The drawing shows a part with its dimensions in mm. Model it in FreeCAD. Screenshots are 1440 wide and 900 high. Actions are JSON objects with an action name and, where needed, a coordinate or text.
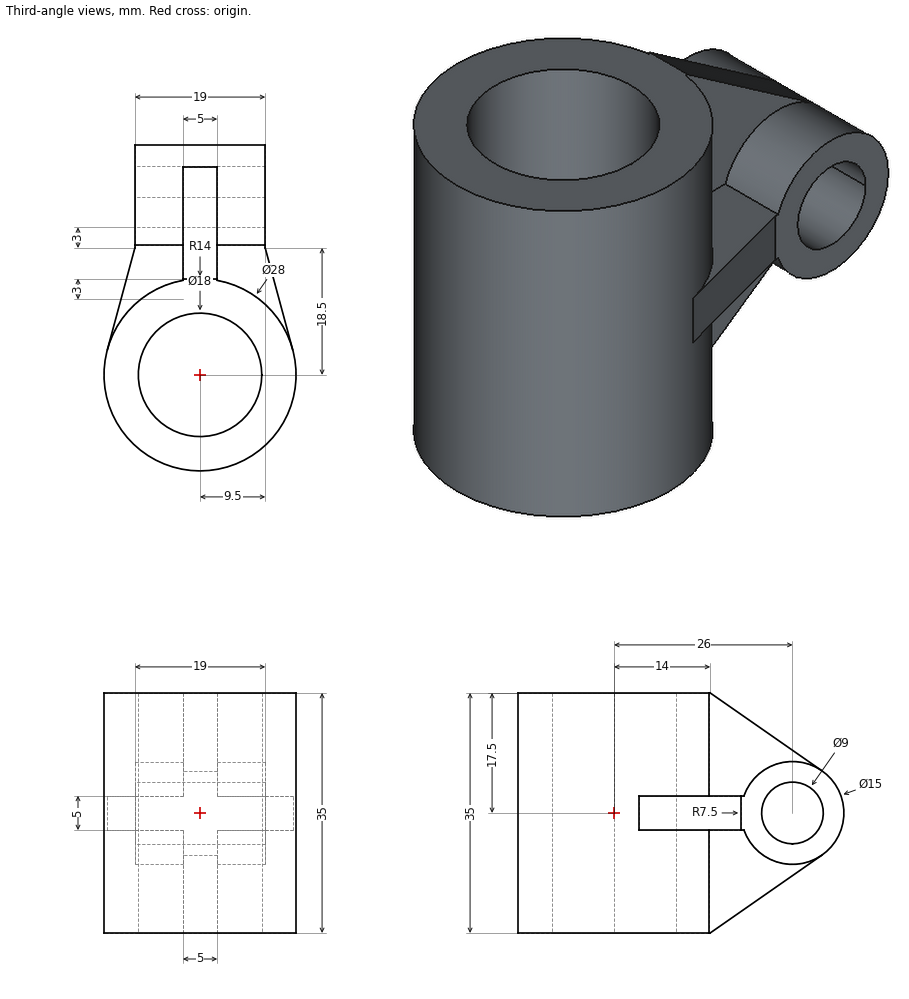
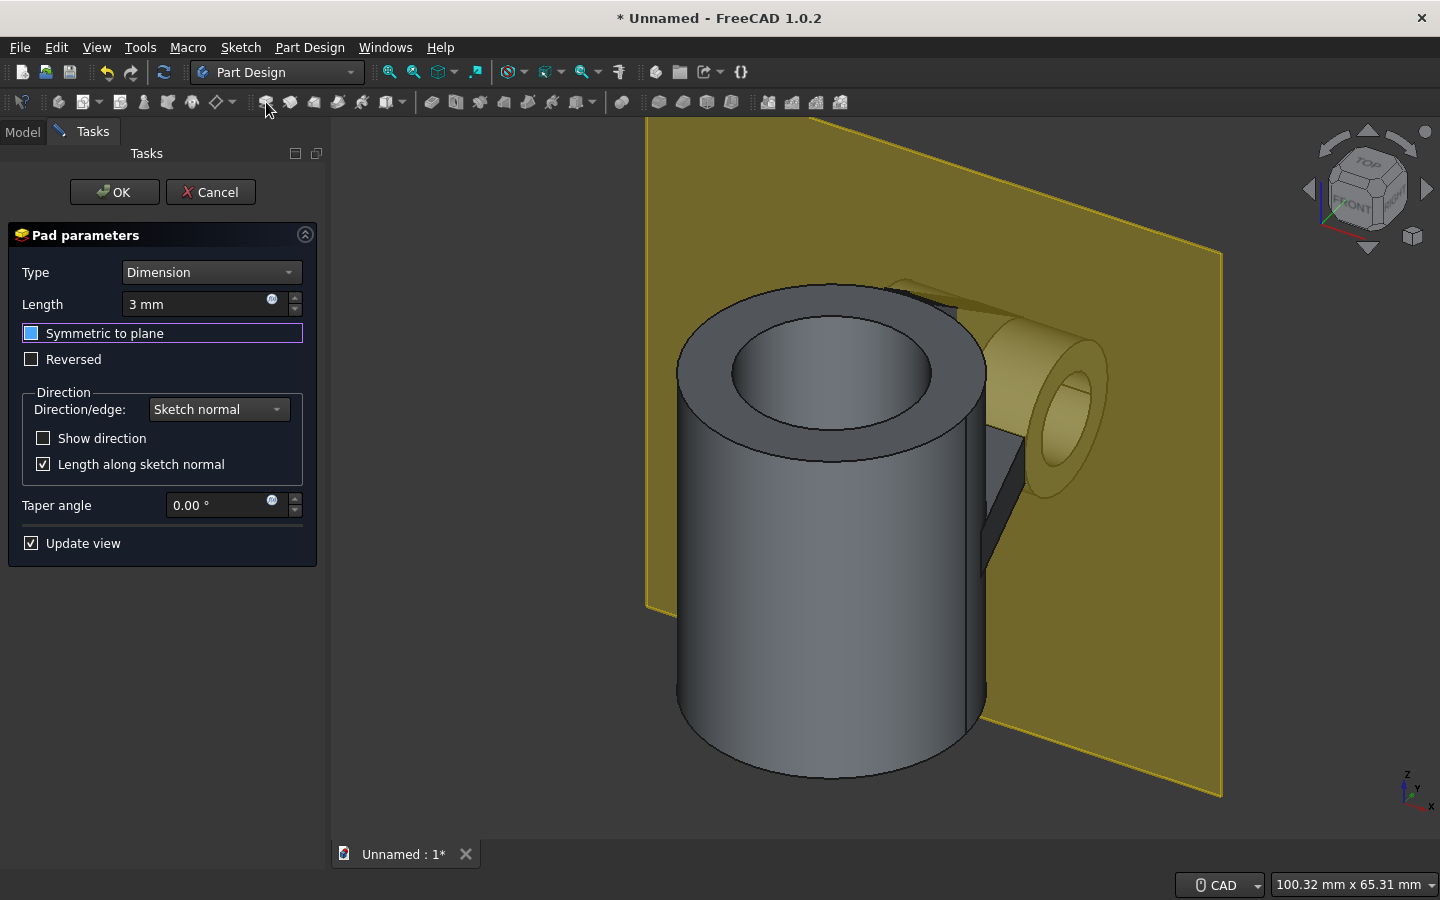
{"action": "left_click", "coordinate": [30, 359]}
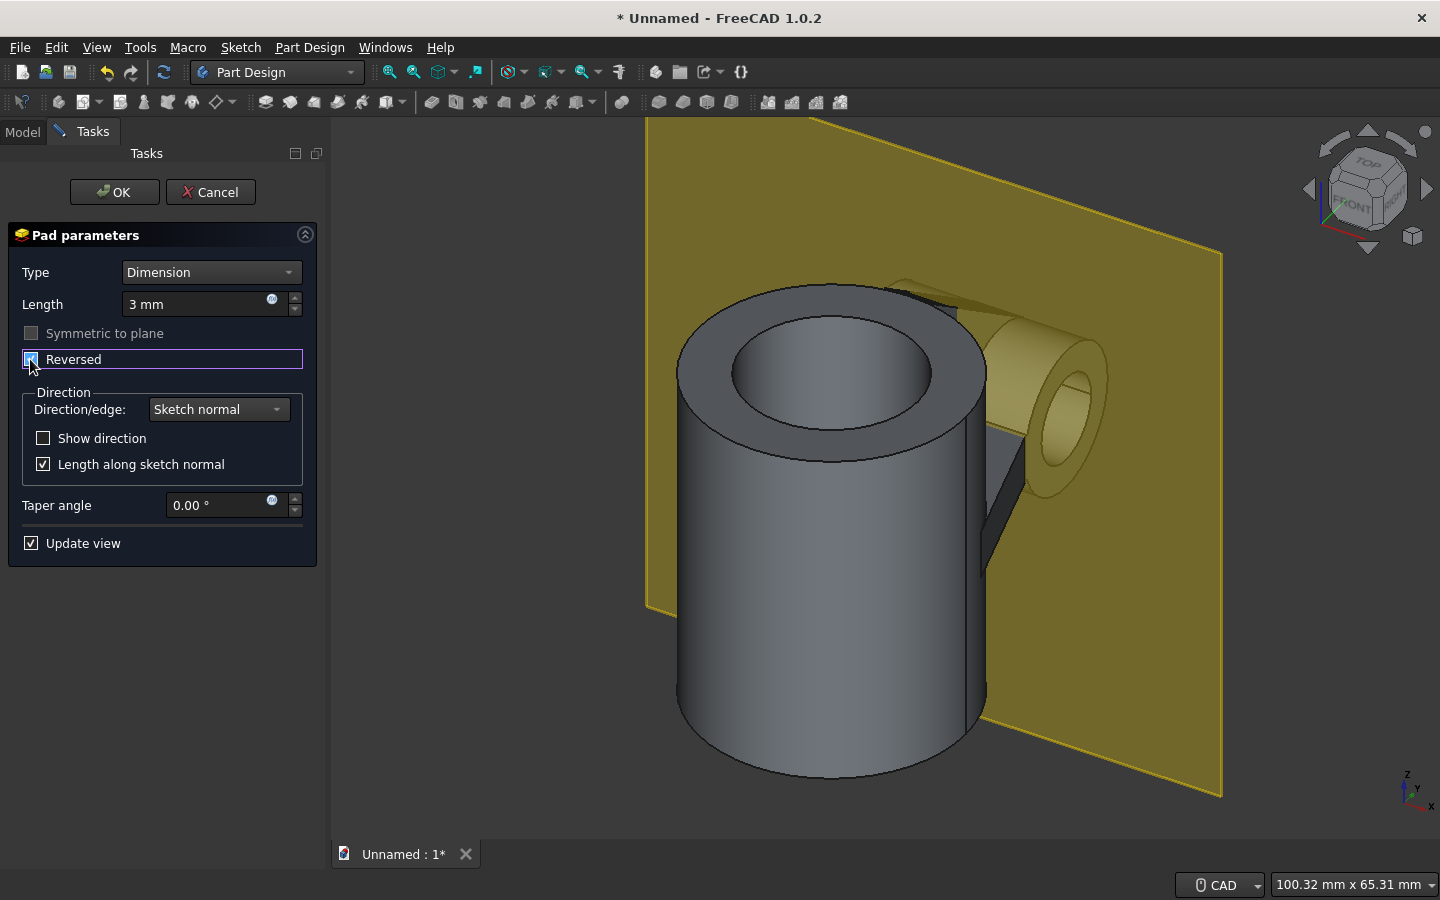
{"action": "left_click", "coordinate": [115, 192]}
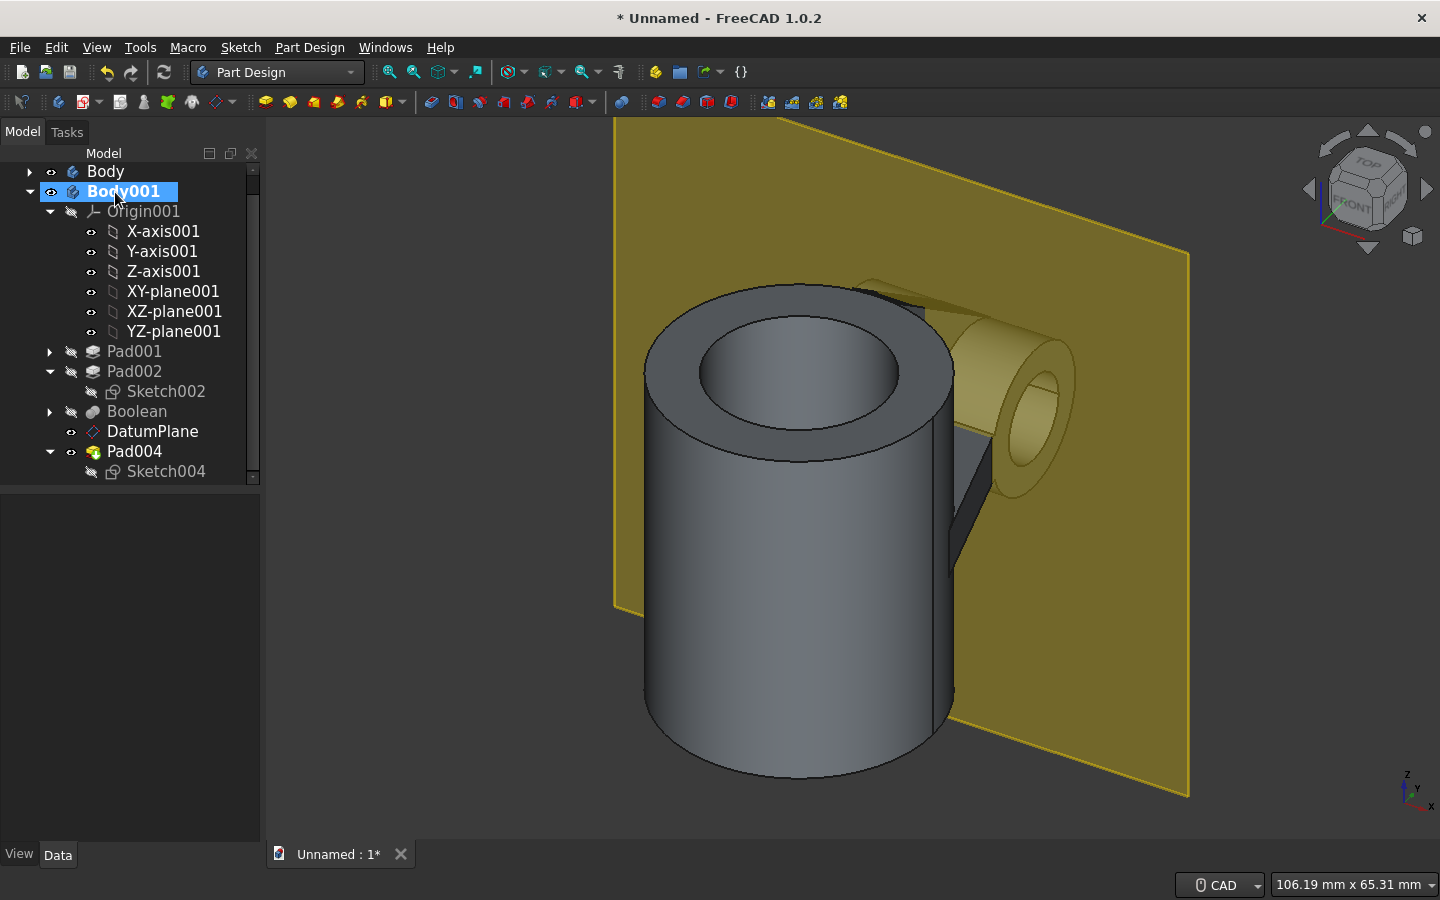
{"action": "left_click", "coordinate": [116, 432]}
{"action": "key", "text": "space"}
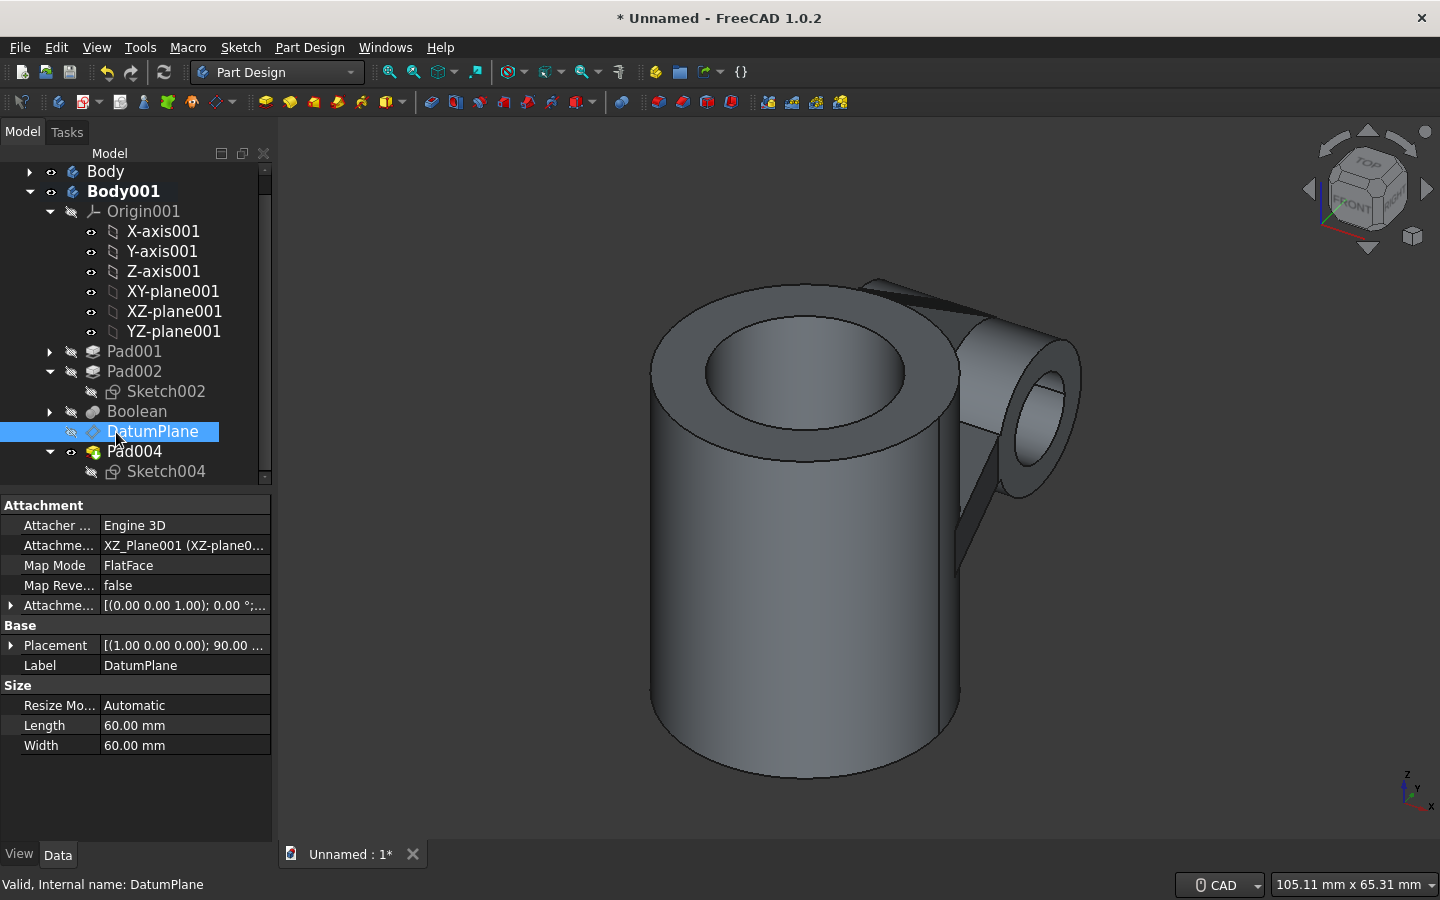
{"action": "double_click", "coordinate": [96, 172]}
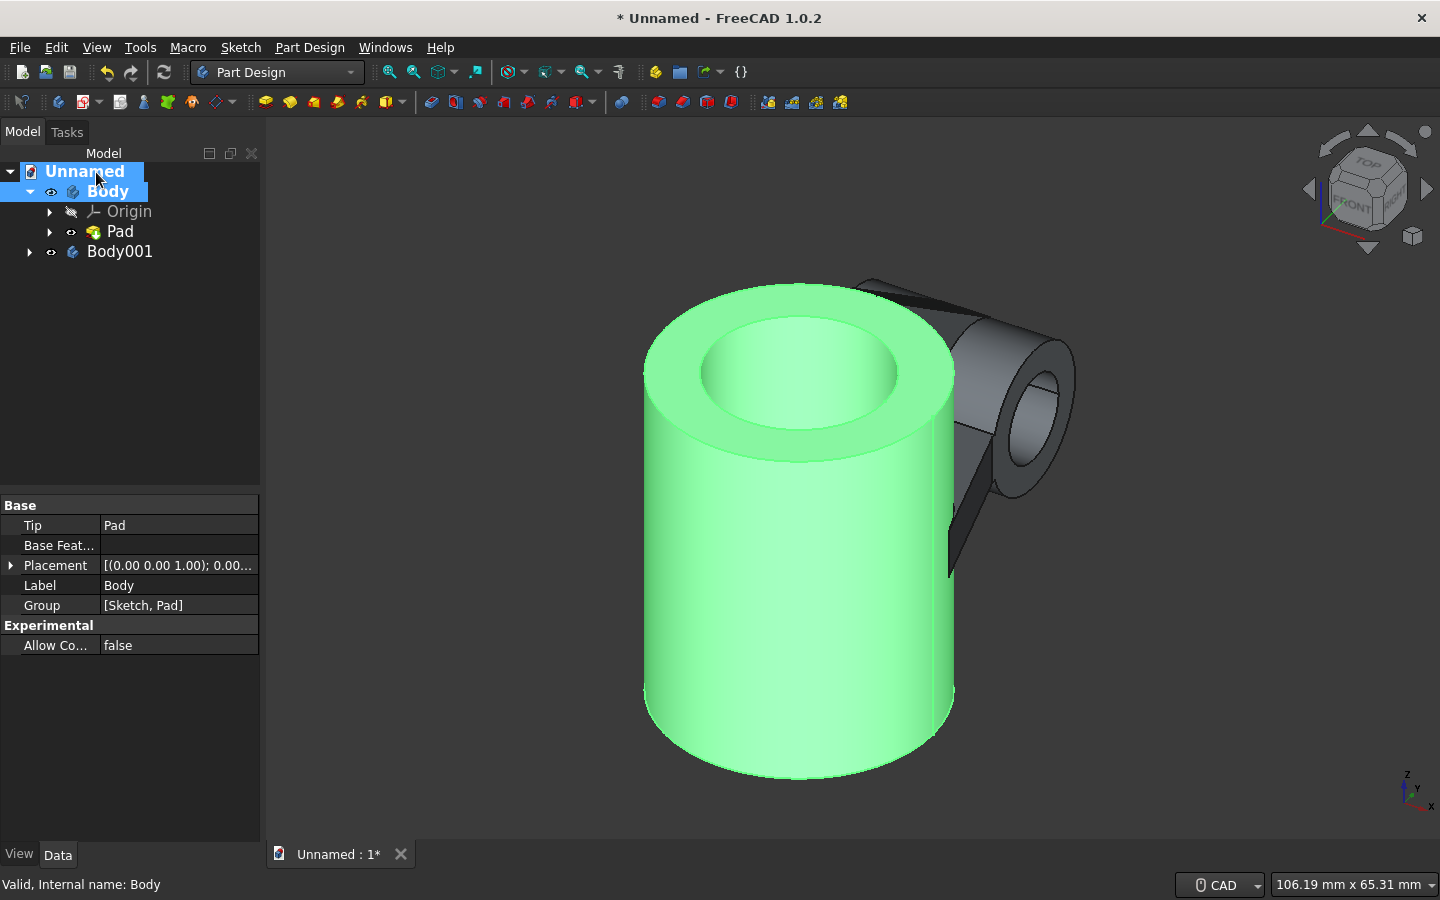
{"action": "left_click", "coordinate": [96, 252]}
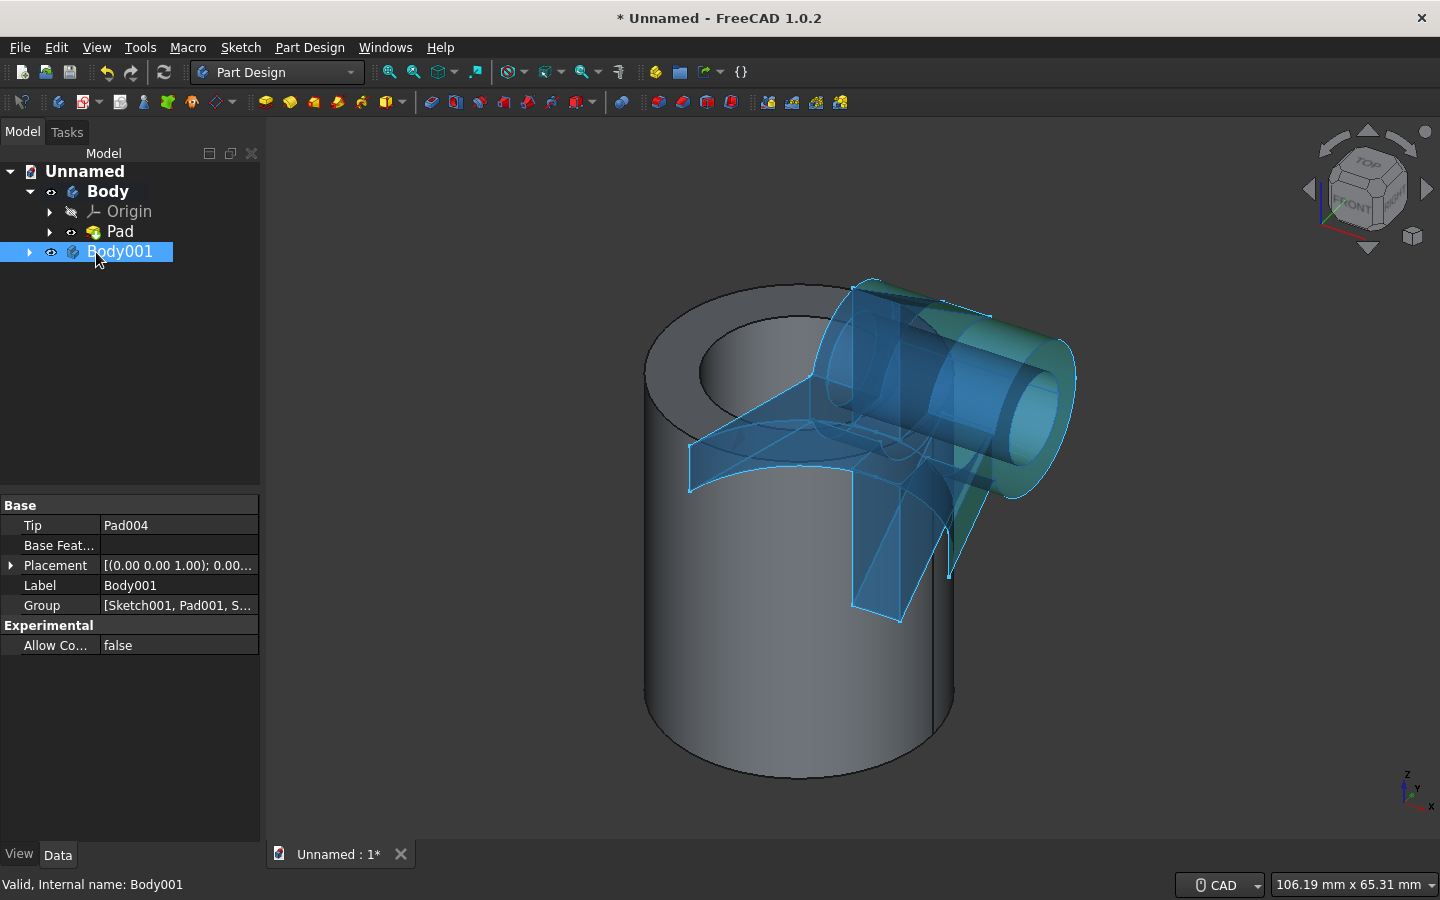
{"action": "left_click", "coordinate": [622, 102]}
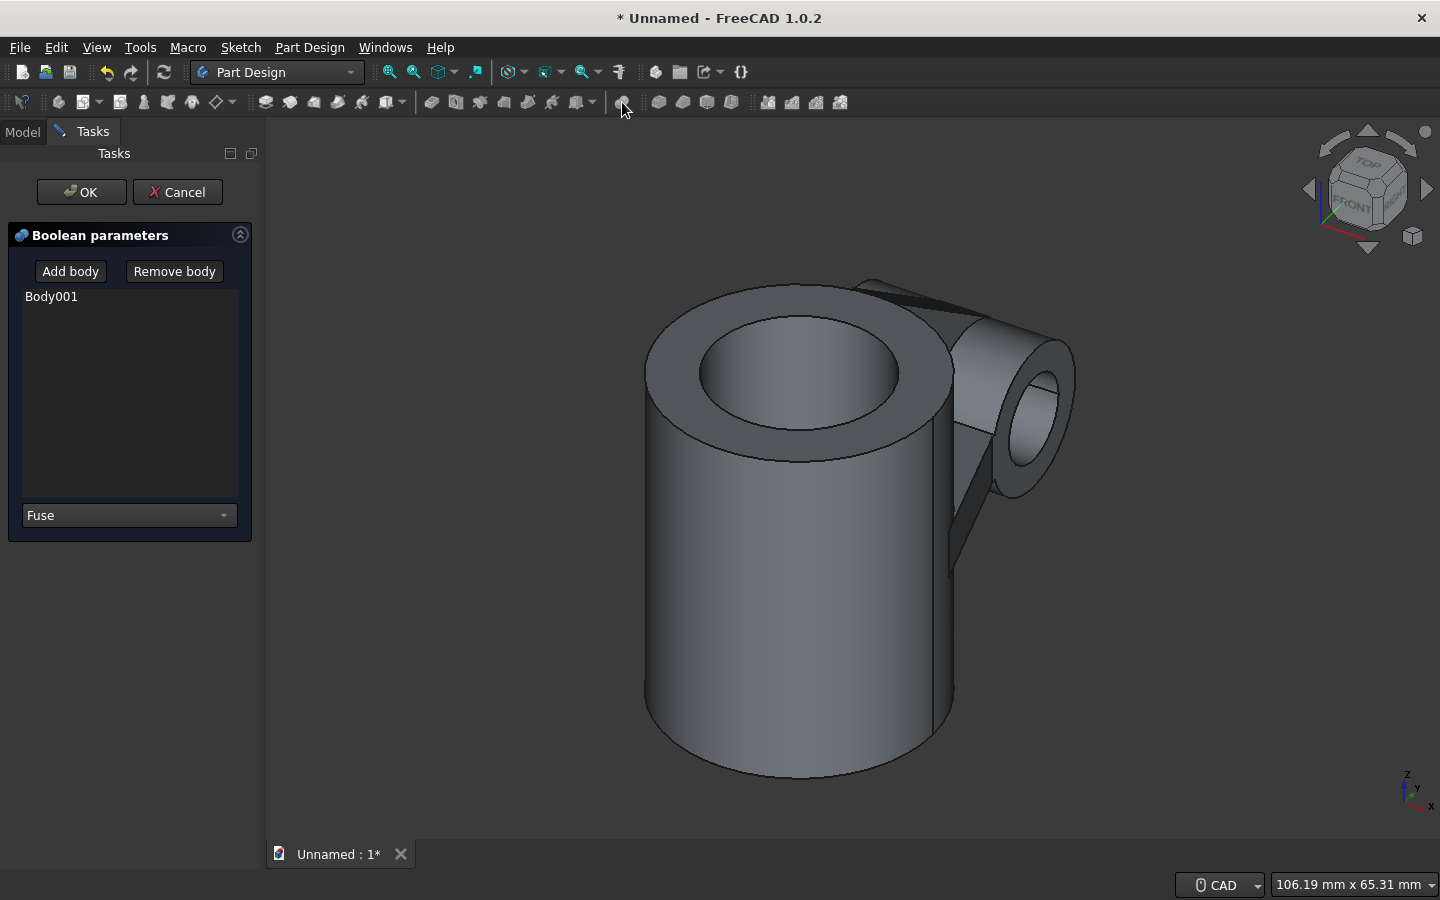
{"action": "left_click", "coordinate": [82, 192]}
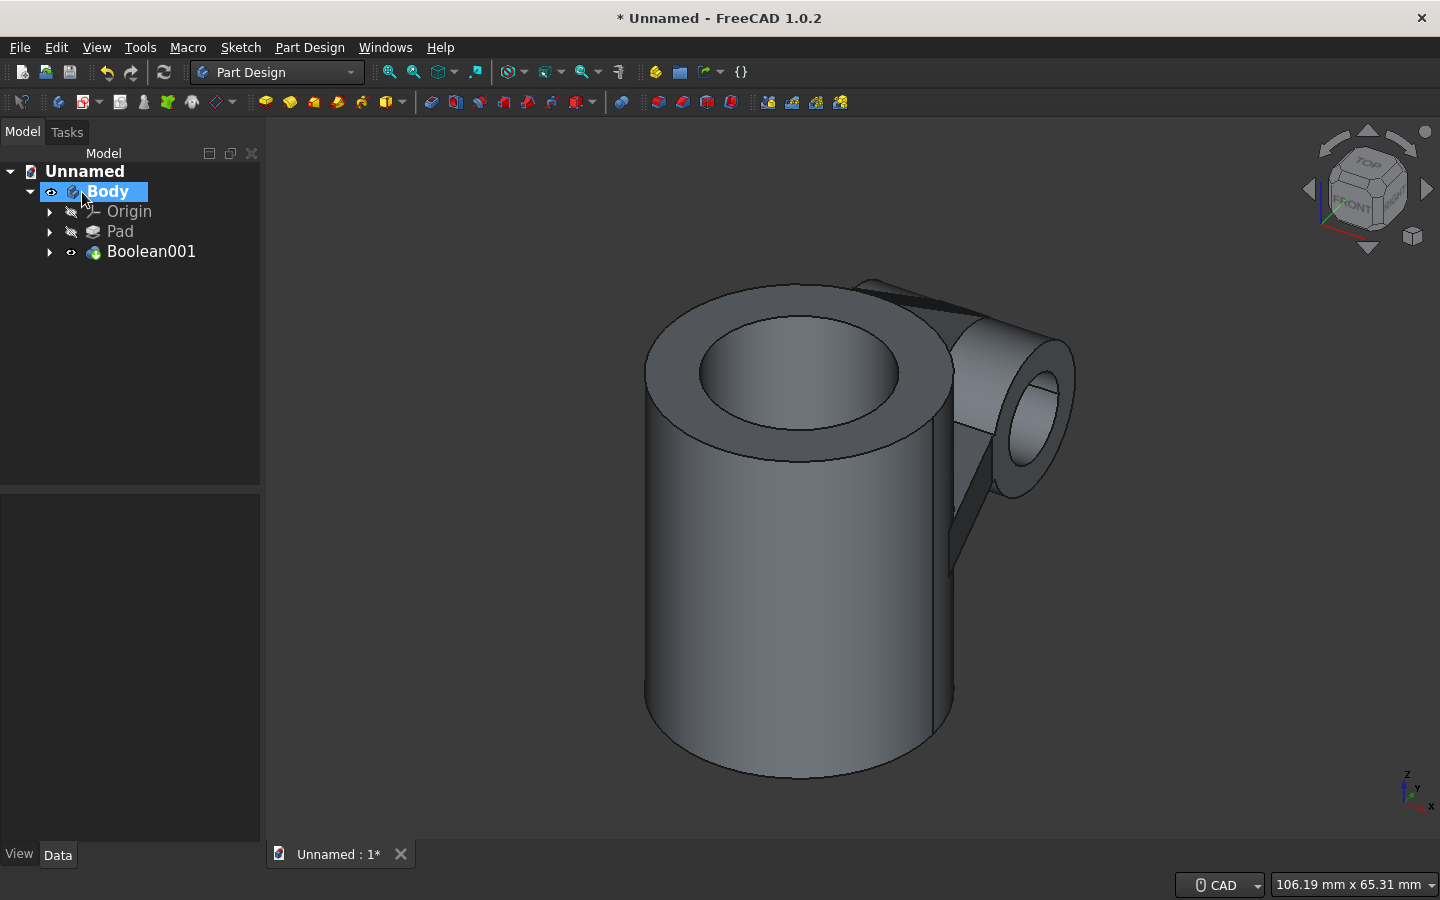
{"action": "left_click", "coordinate": [50, 212]}